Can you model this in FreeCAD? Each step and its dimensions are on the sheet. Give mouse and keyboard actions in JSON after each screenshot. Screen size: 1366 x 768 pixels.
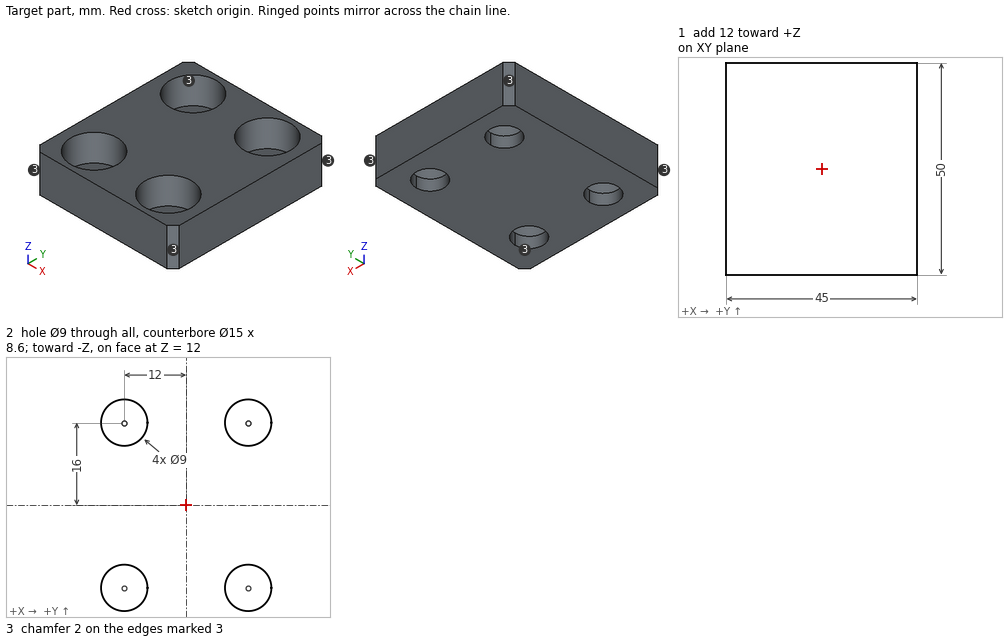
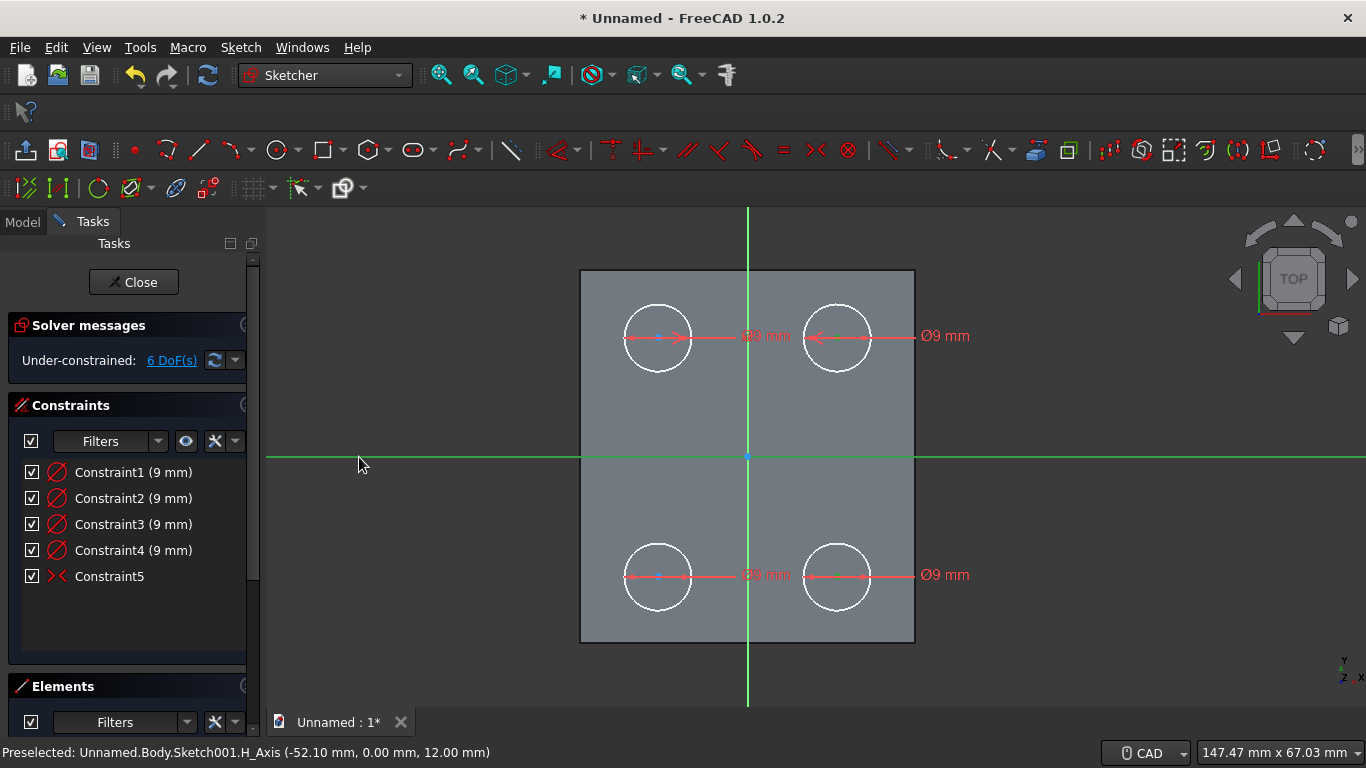
{"action": "left_click", "coordinate": [816, 150]}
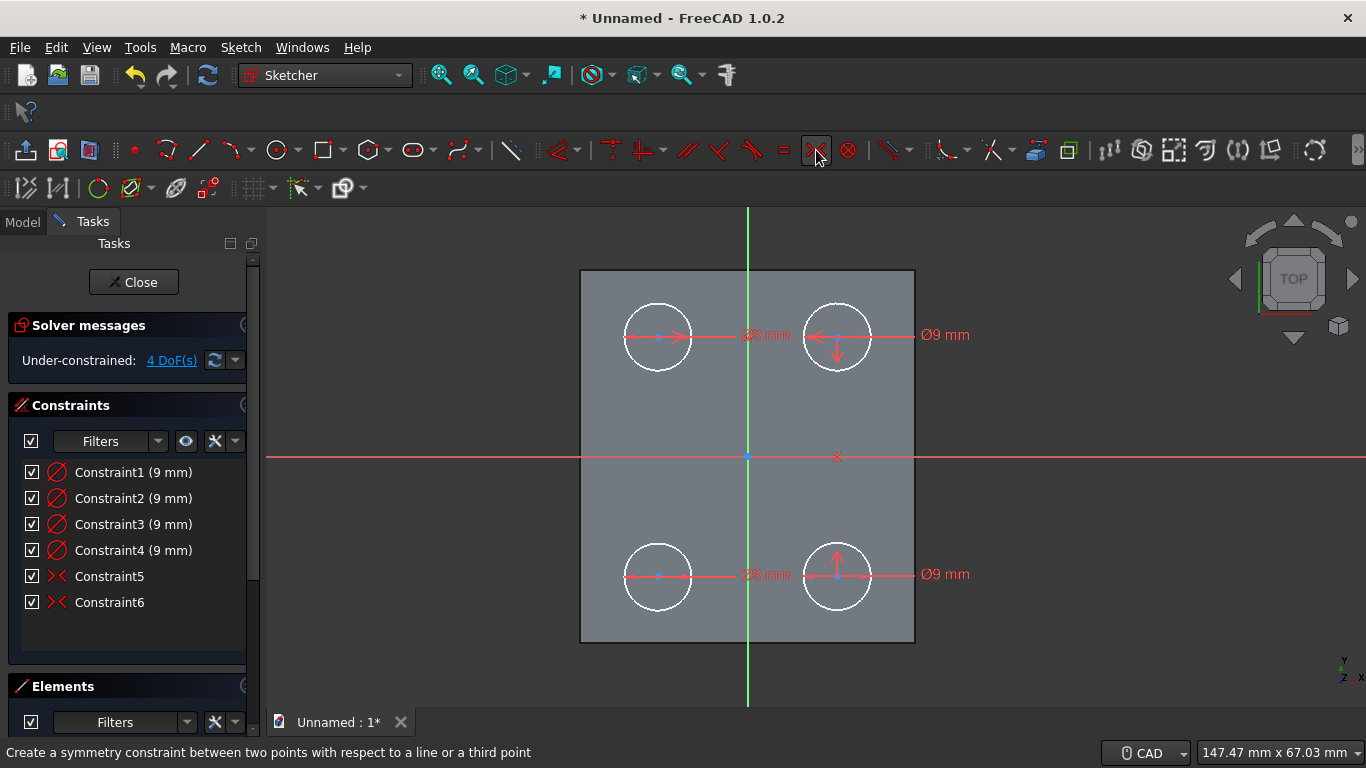
{"action": "left_click", "coordinate": [658, 337]}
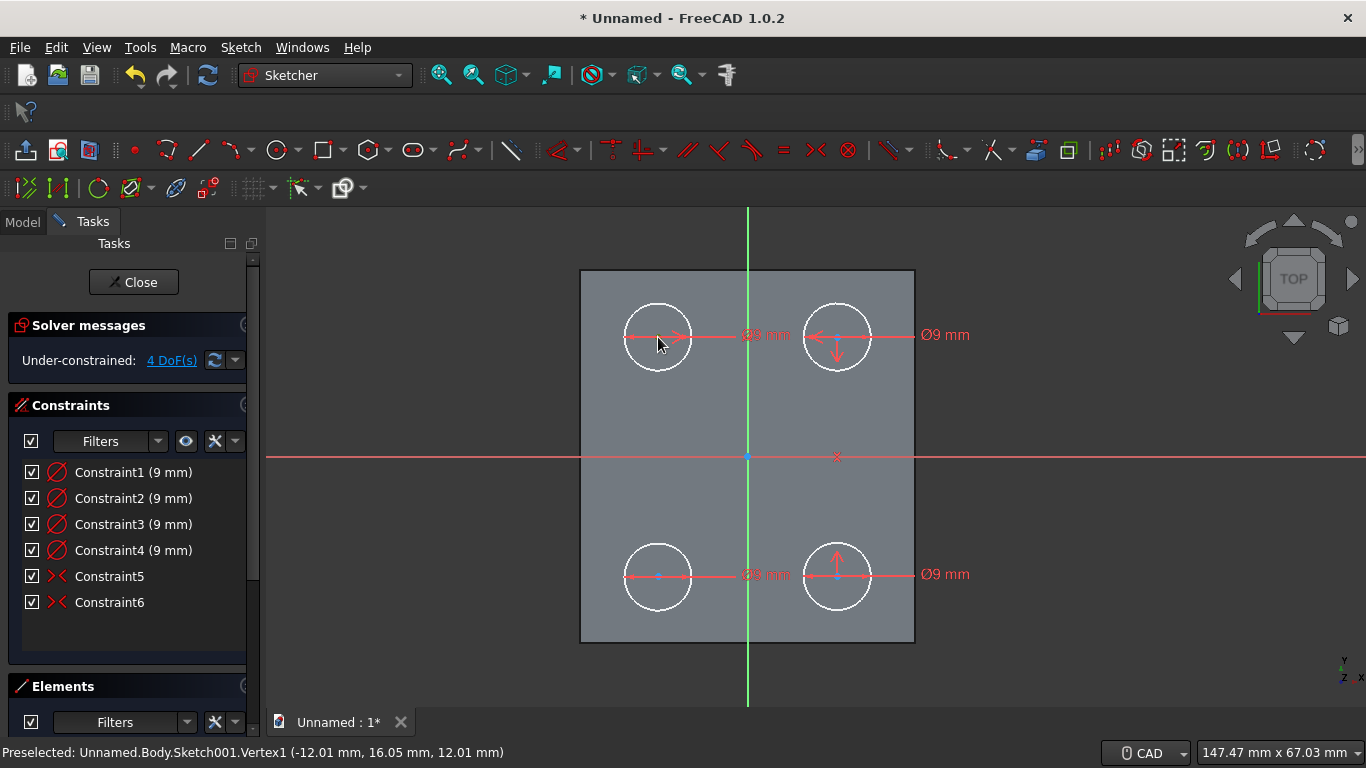
{"action": "left_click", "coordinate": [658, 577]}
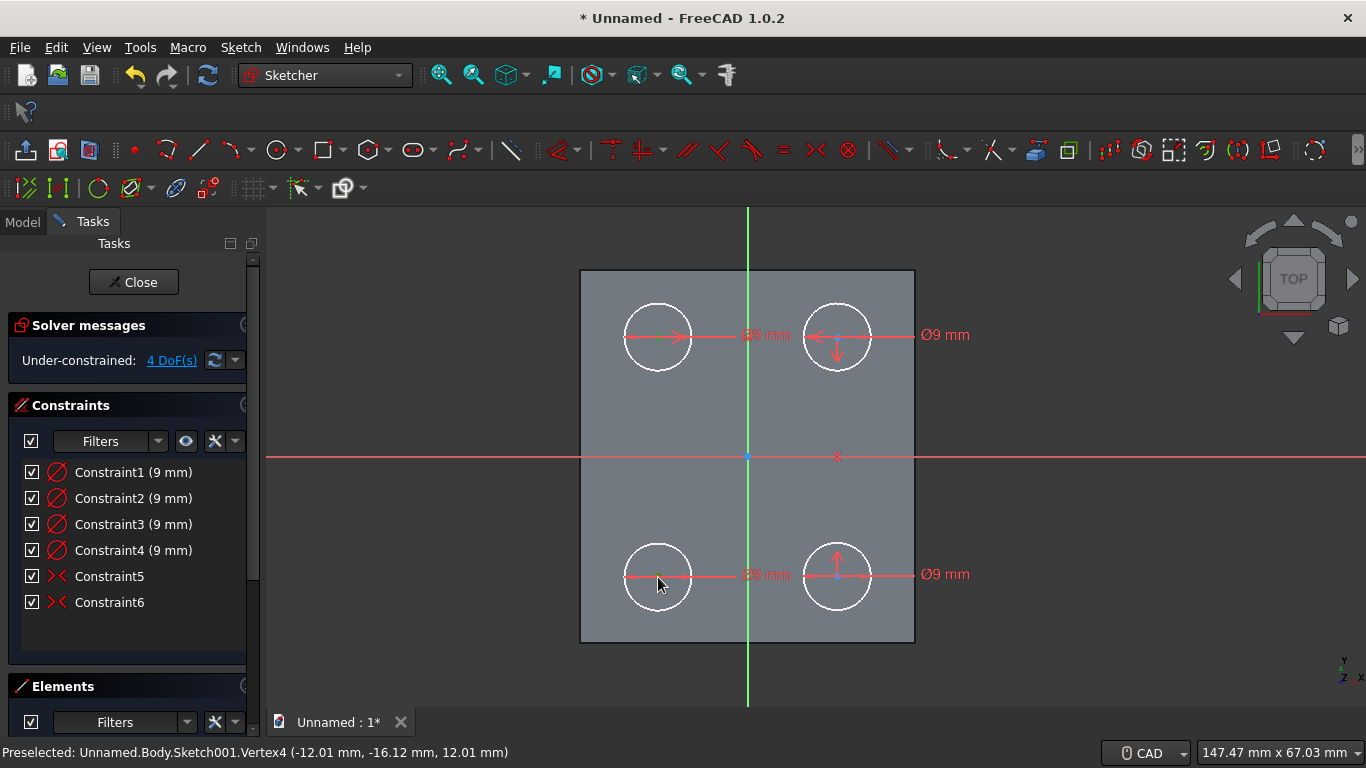
{"action": "left_click", "coordinate": [359, 457]}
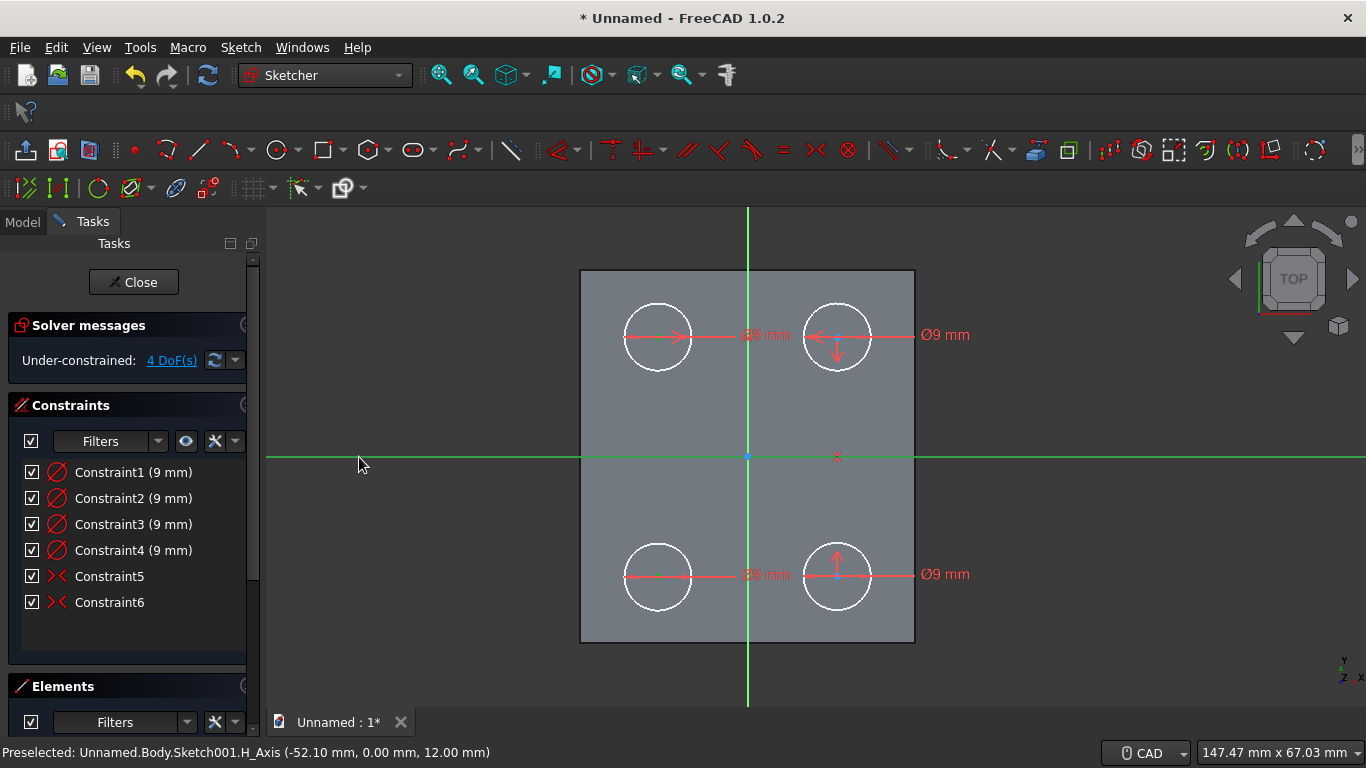
{"action": "left_click", "coordinate": [816, 150]}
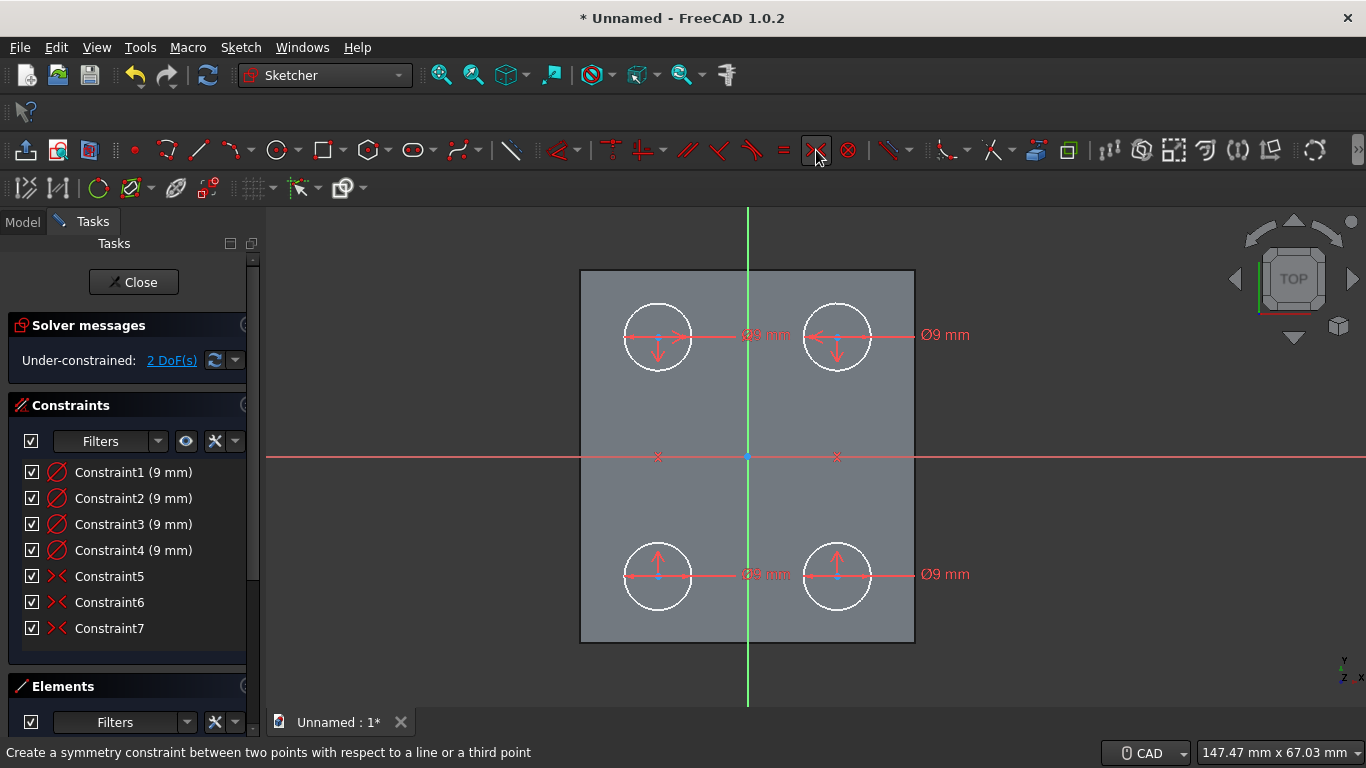
{"action": "left_click", "coordinate": [558, 150]}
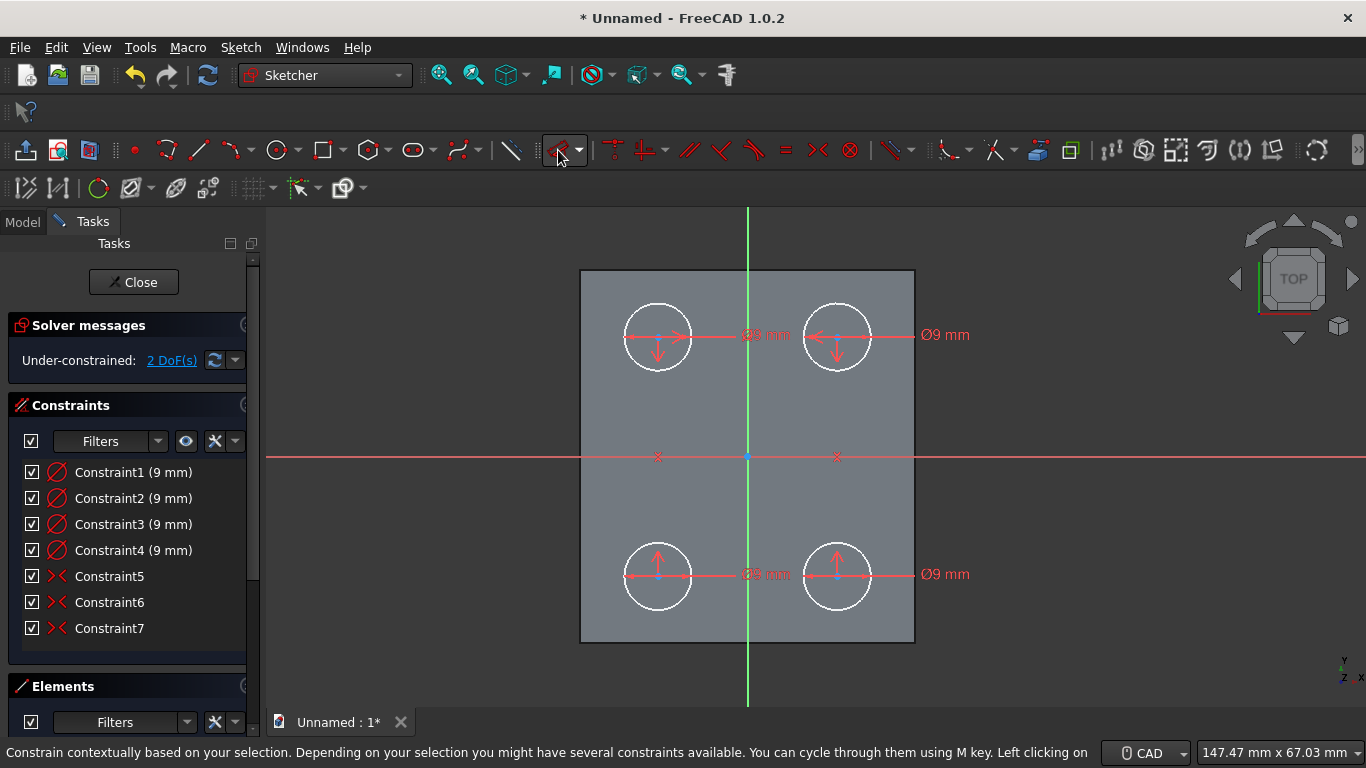
{"action": "left_click", "coordinate": [658, 337]}
{"action": "left_click", "coordinate": [703, 303]}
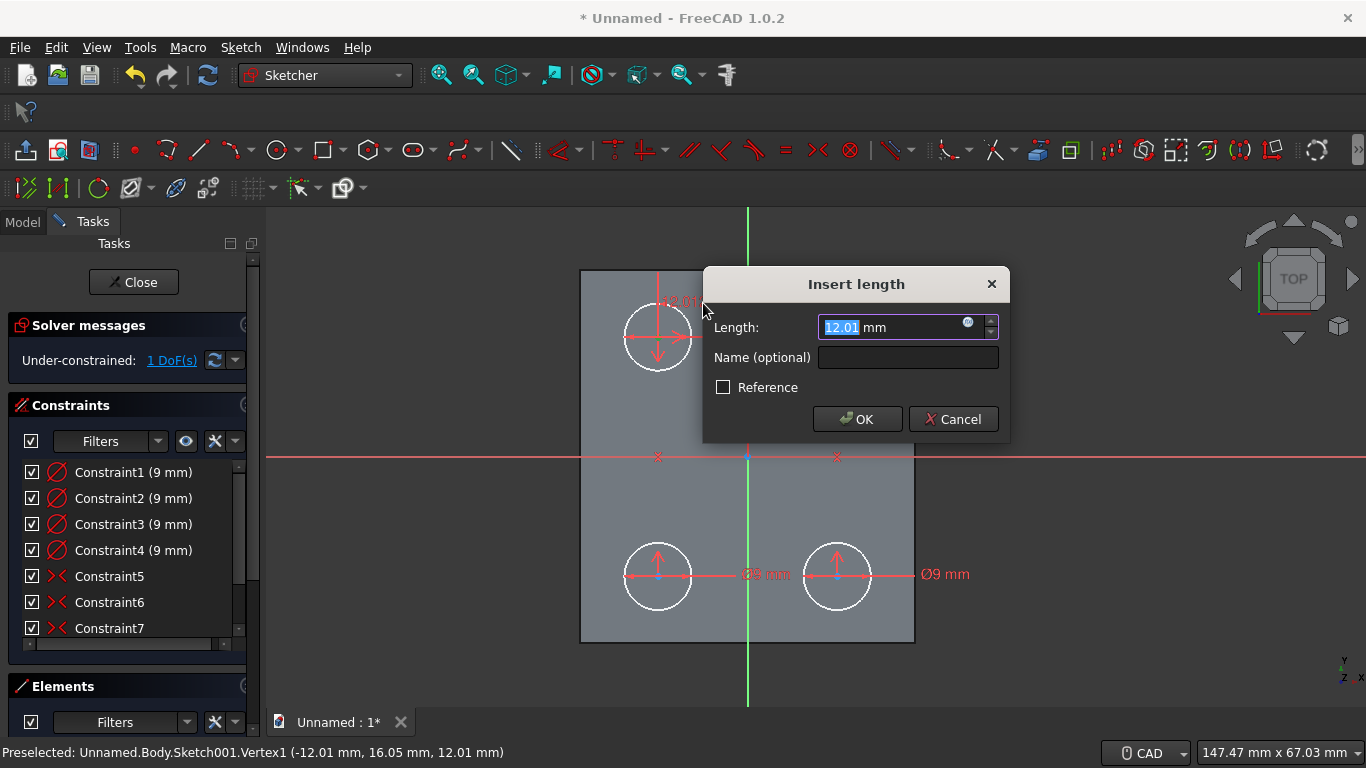
{"action": "type", "text": "12"}
{"action": "key", "text": "Return"}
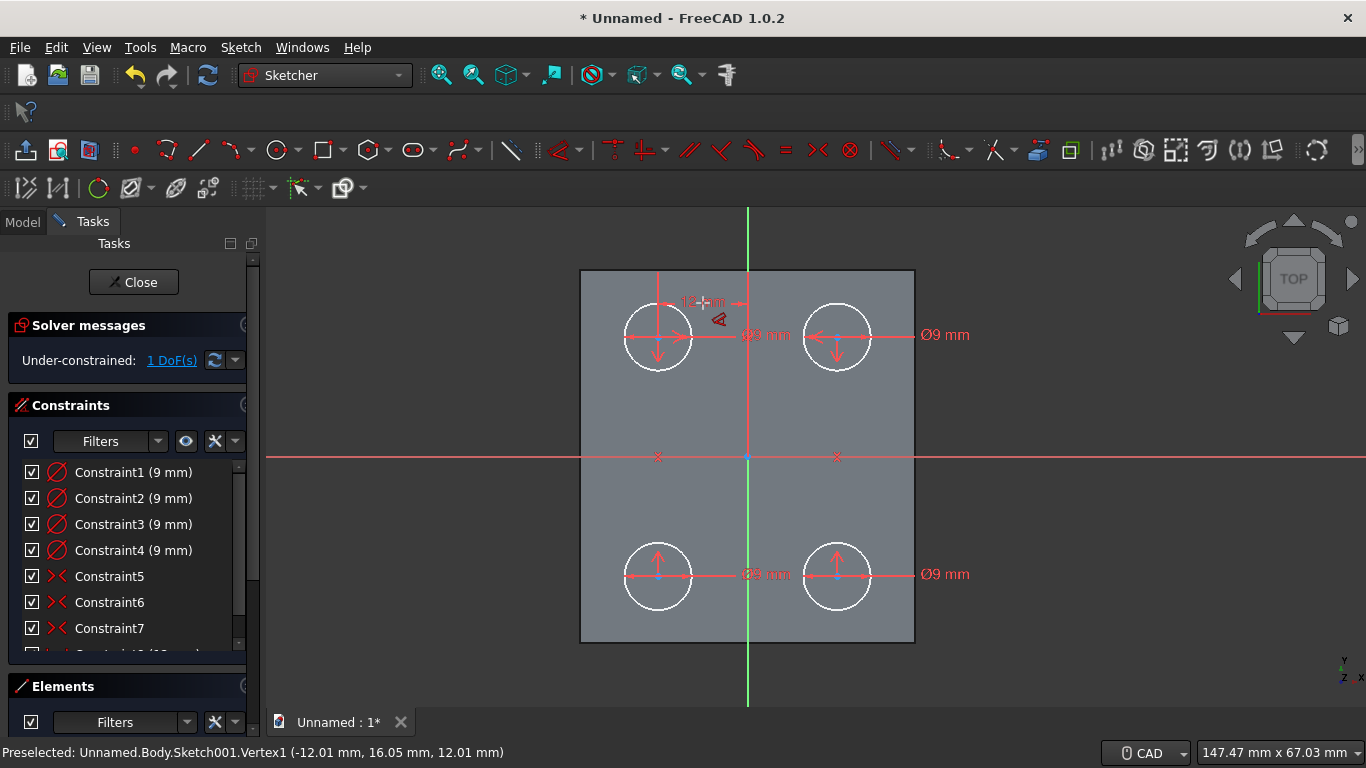
{"action": "left_click", "coordinate": [658, 337]}
{"action": "left_click", "coordinate": [624, 397]}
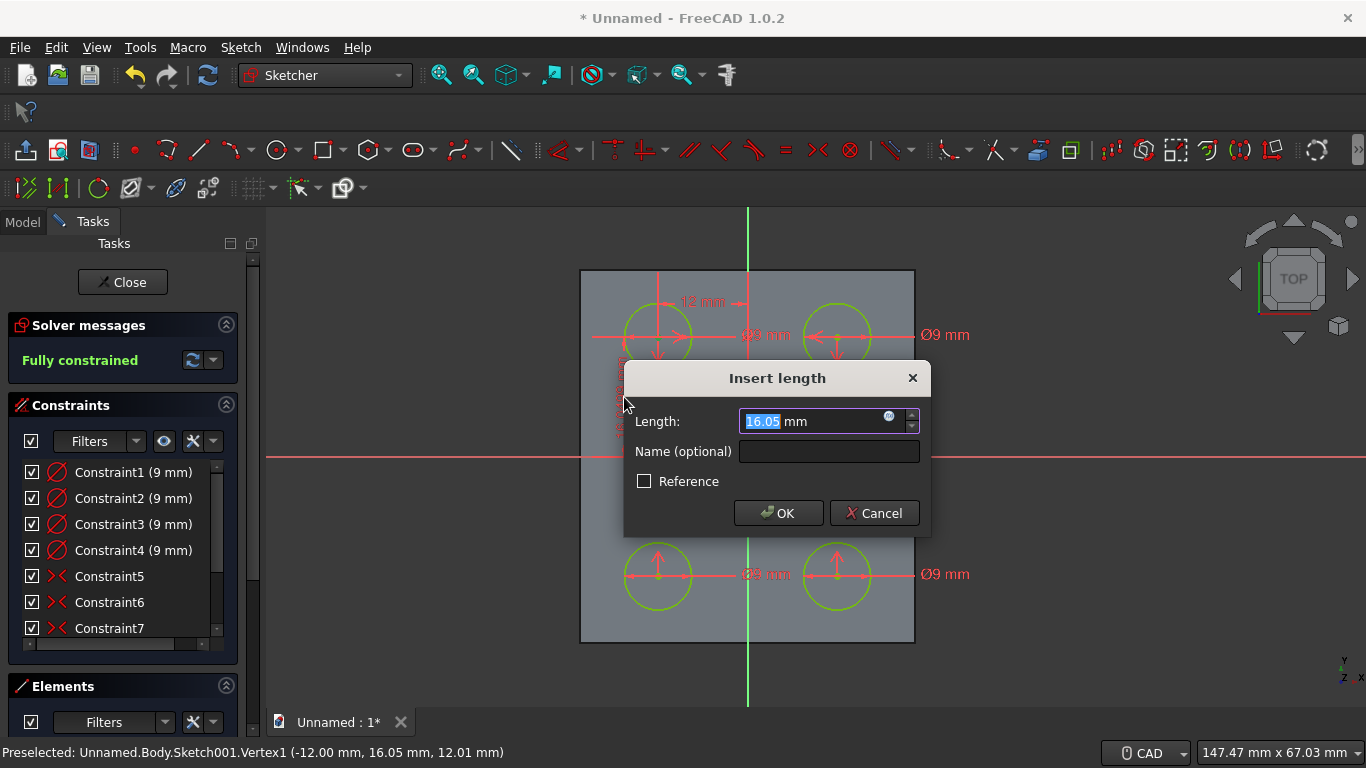
{"action": "type", "text": "16"}
{"action": "key", "text": "Return"}
{"action": "key", "text": "Escape"}